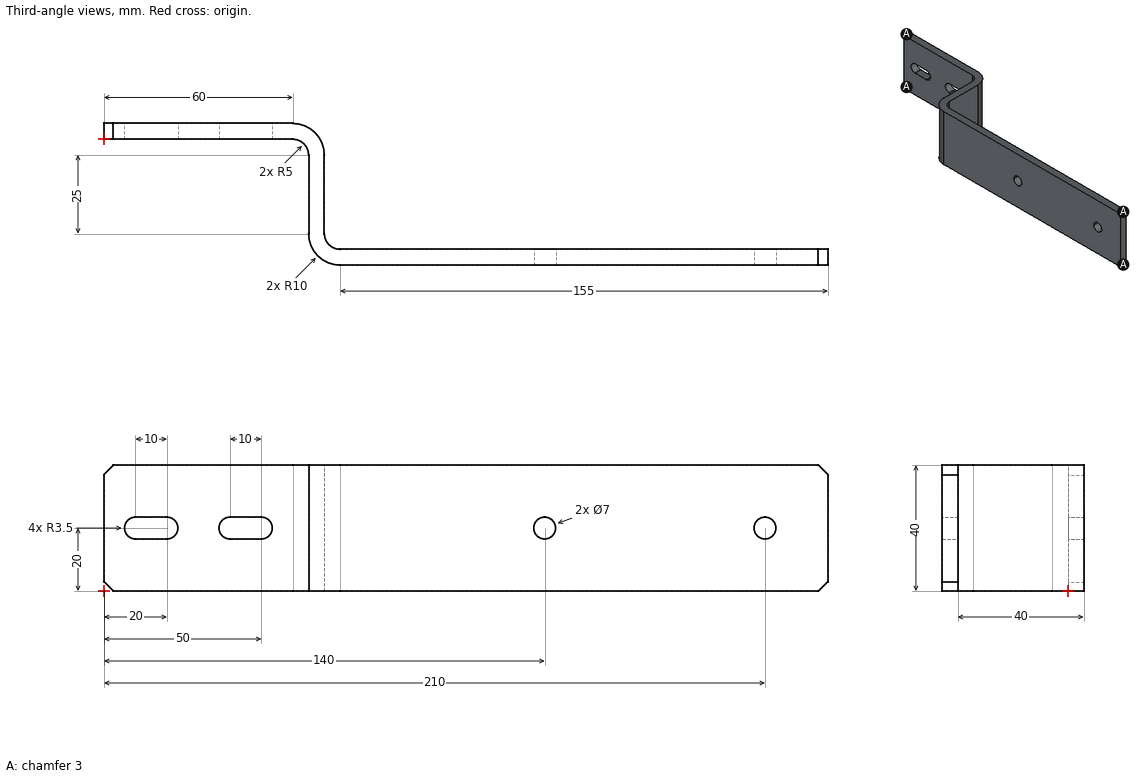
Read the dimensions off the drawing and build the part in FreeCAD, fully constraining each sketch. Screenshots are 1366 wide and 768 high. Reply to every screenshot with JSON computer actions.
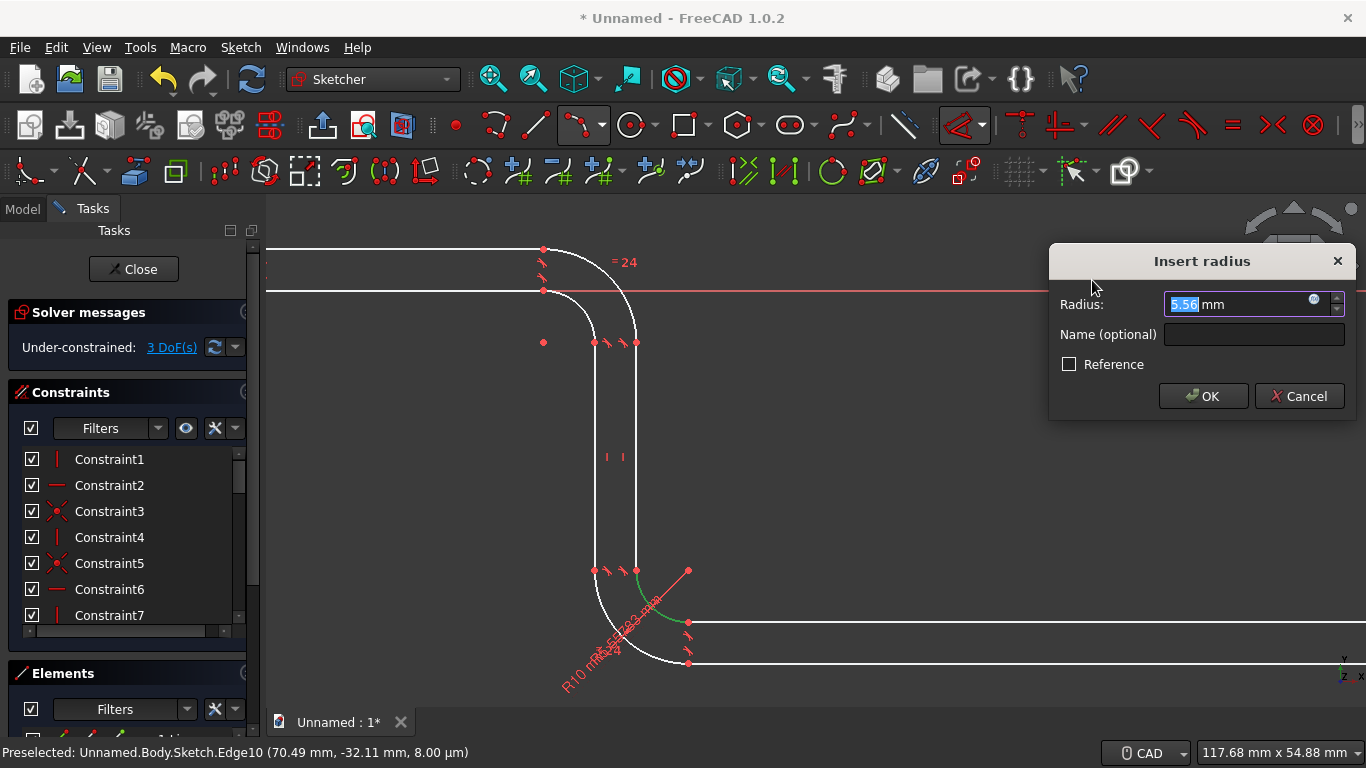
{"action": "type", "text": "5"}
{"action": "key", "text": "Return"}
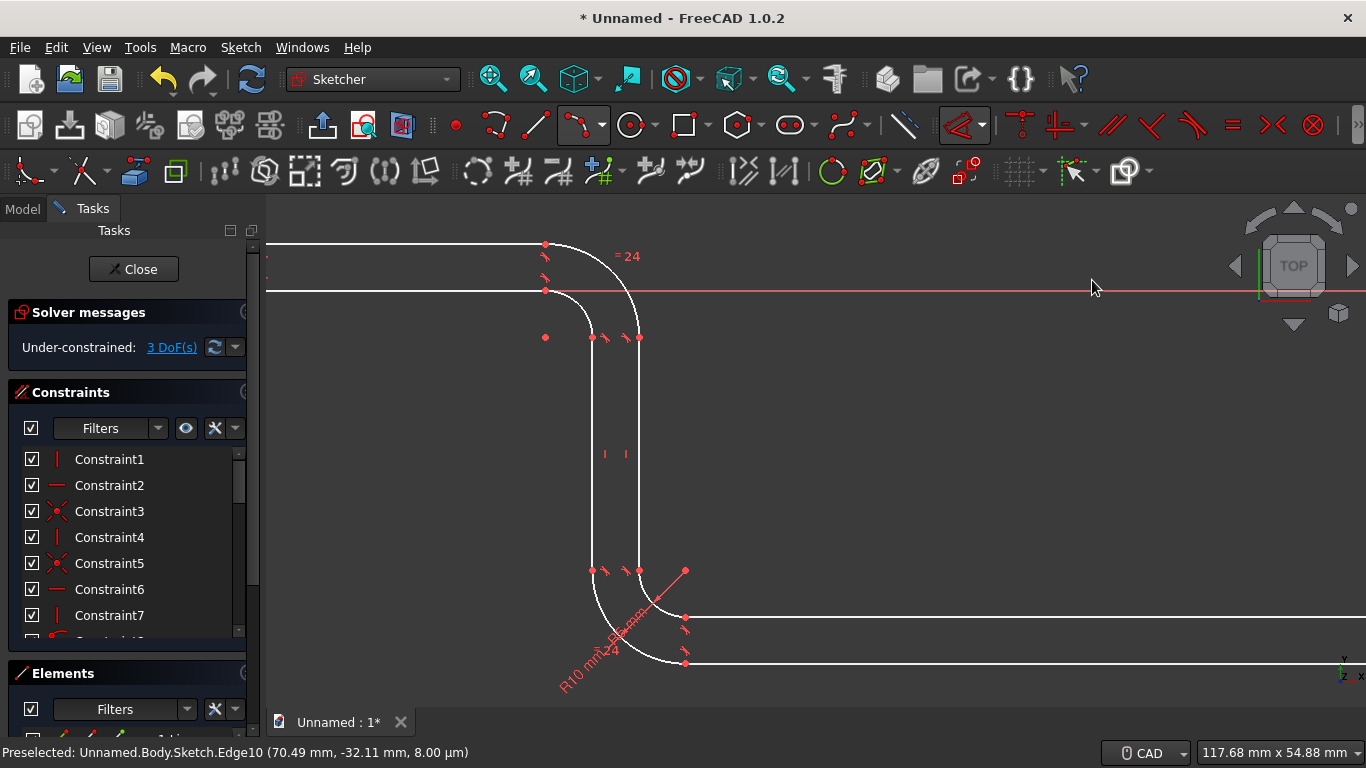
{"action": "scroll", "coordinate": [614, 449], "scroll_direction": "down", "scroll_amount": 6}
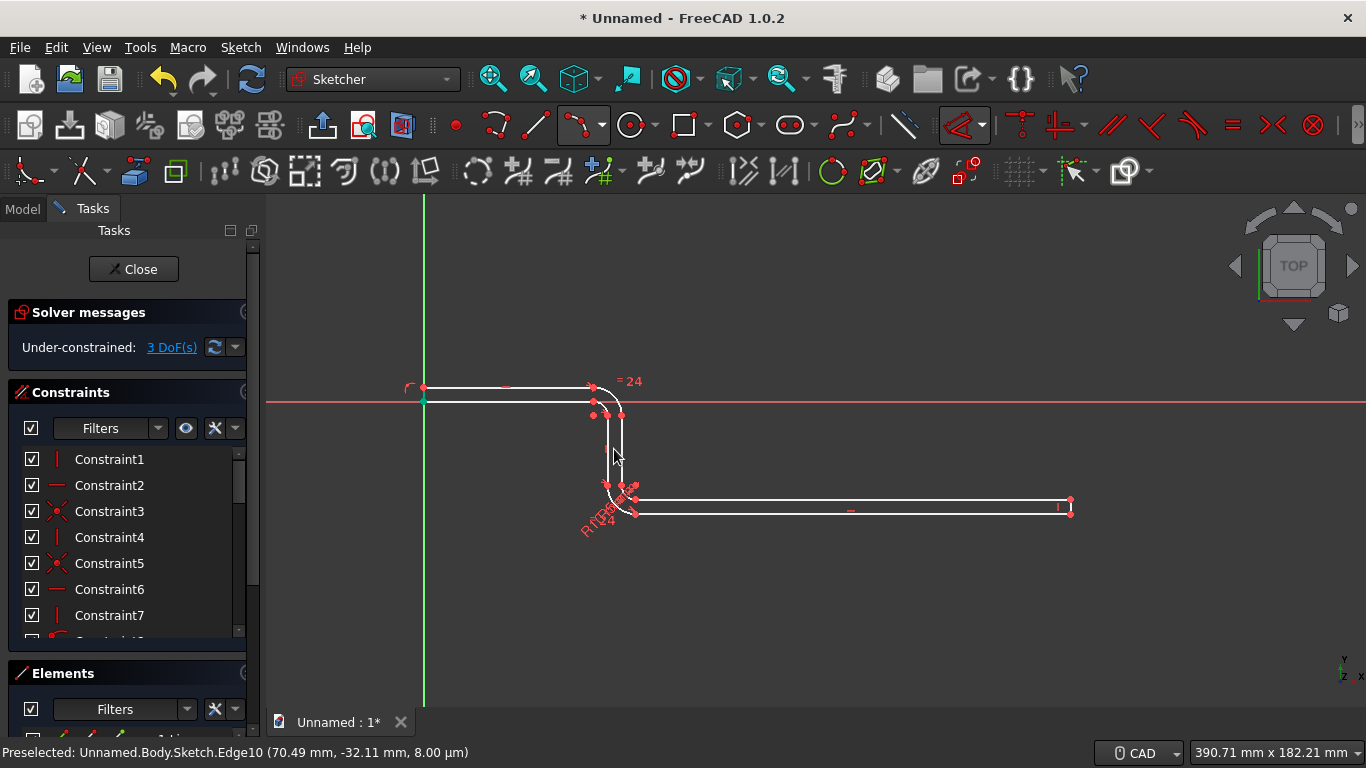
{"action": "left_click", "coordinate": [608, 437]}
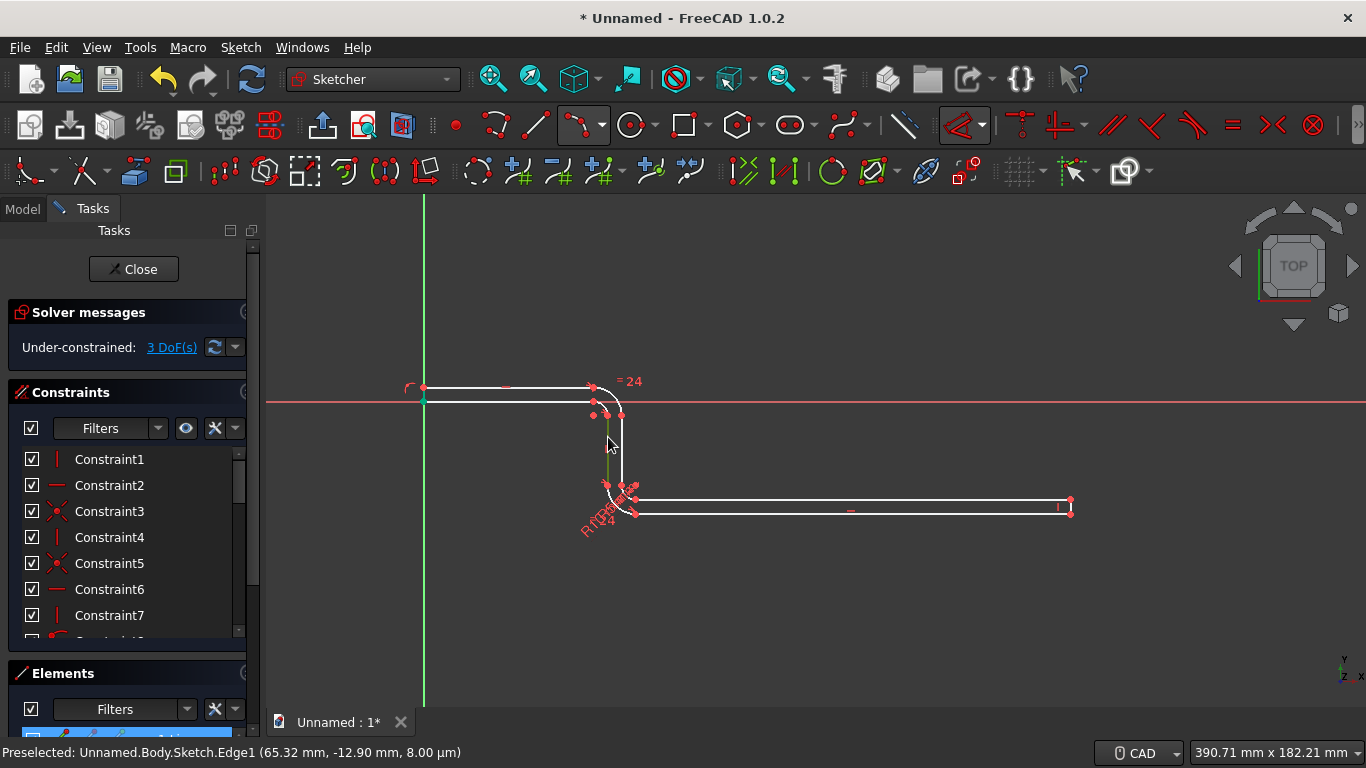
{"action": "key", "text": "i"}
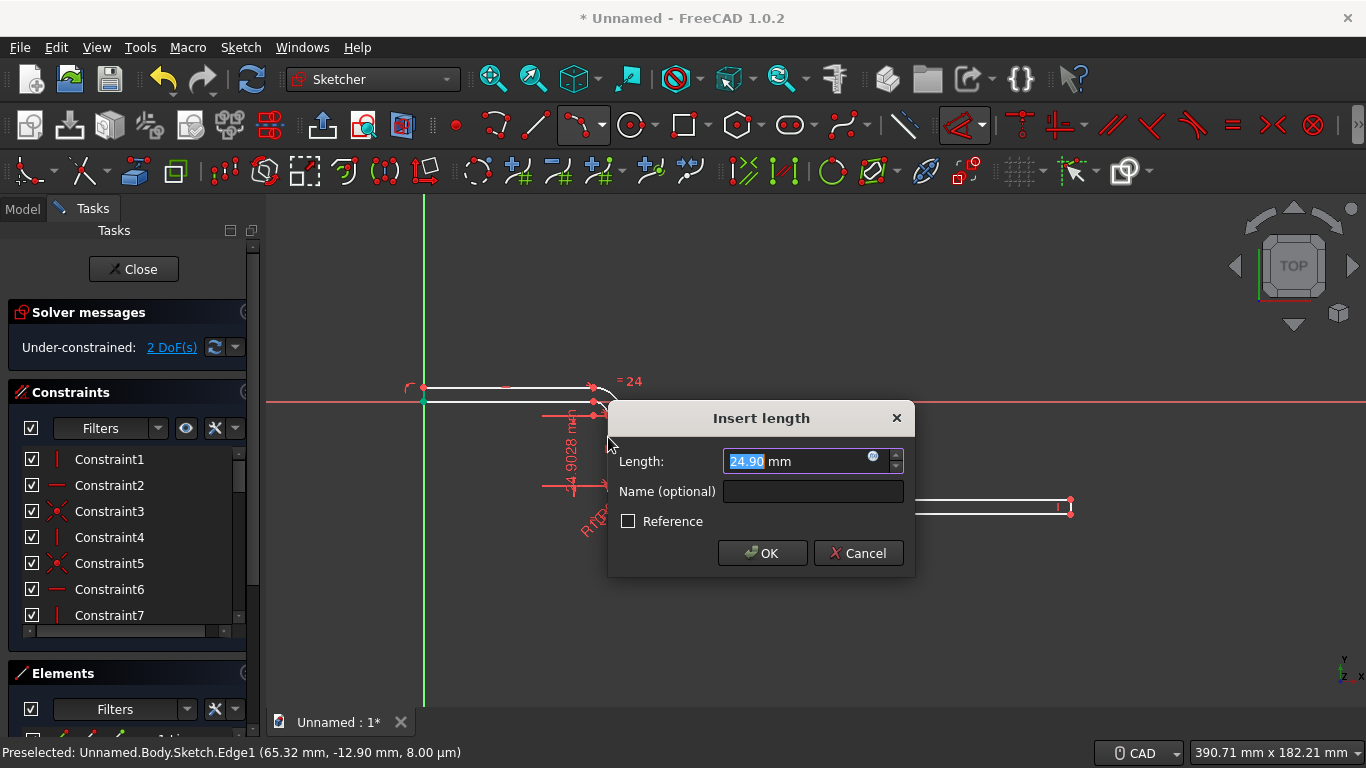
{"action": "type", "text": "25"}
{"action": "key", "text": "Return"}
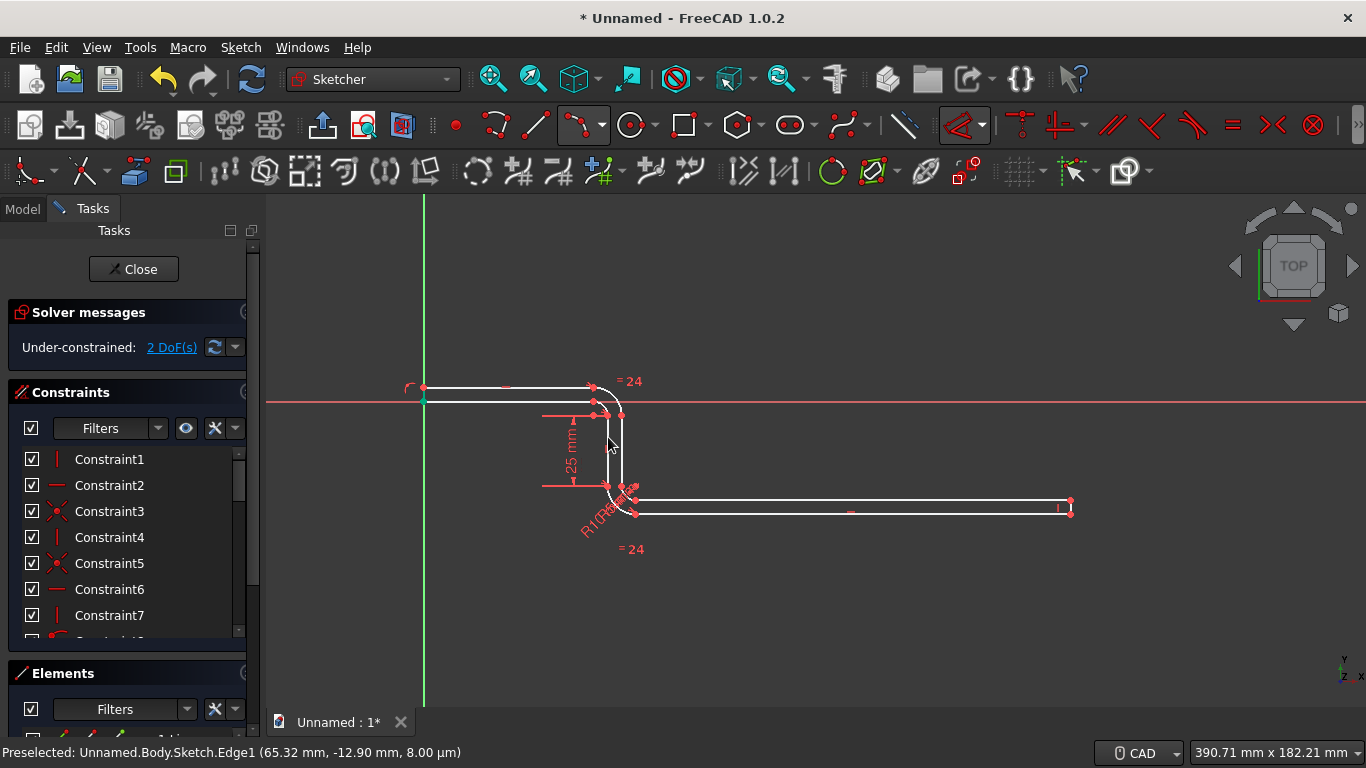
{"action": "left_click", "coordinate": [543, 388]}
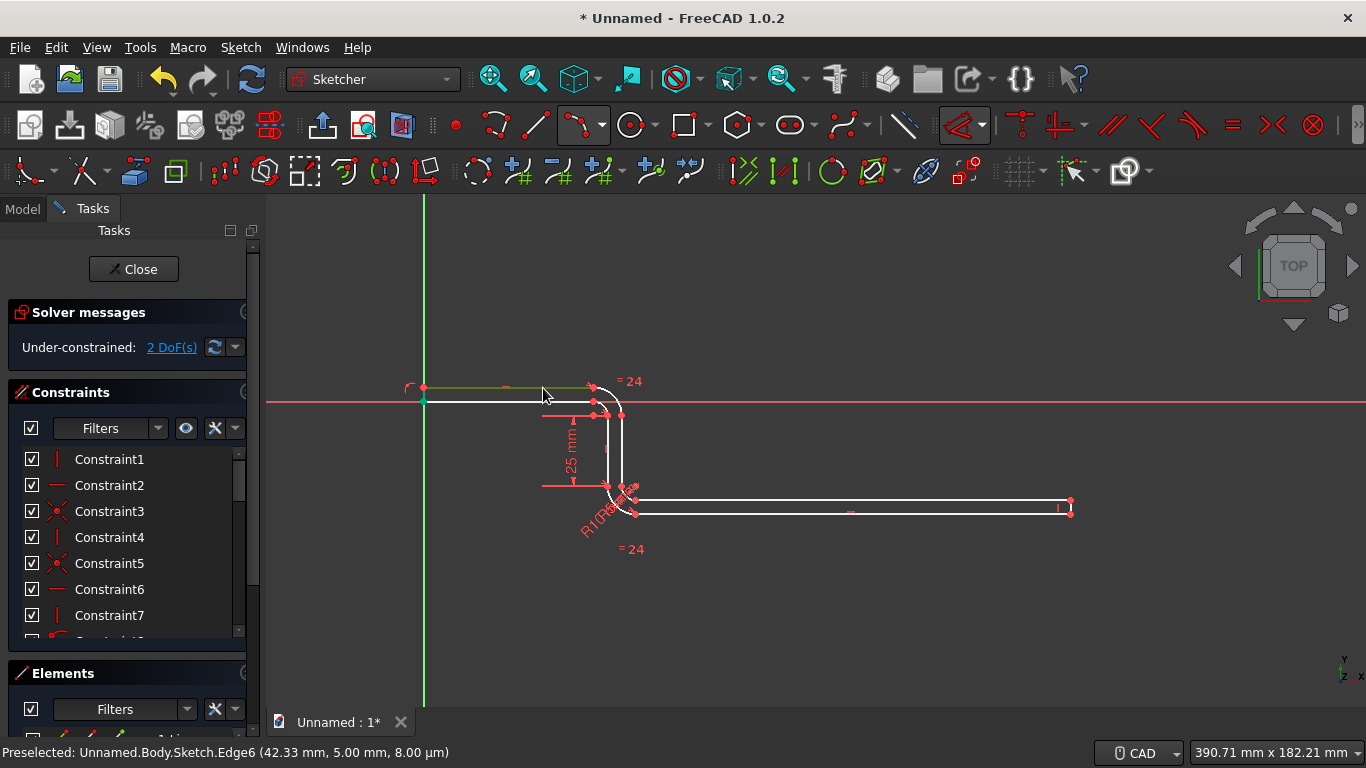
{"action": "key", "text": "l"}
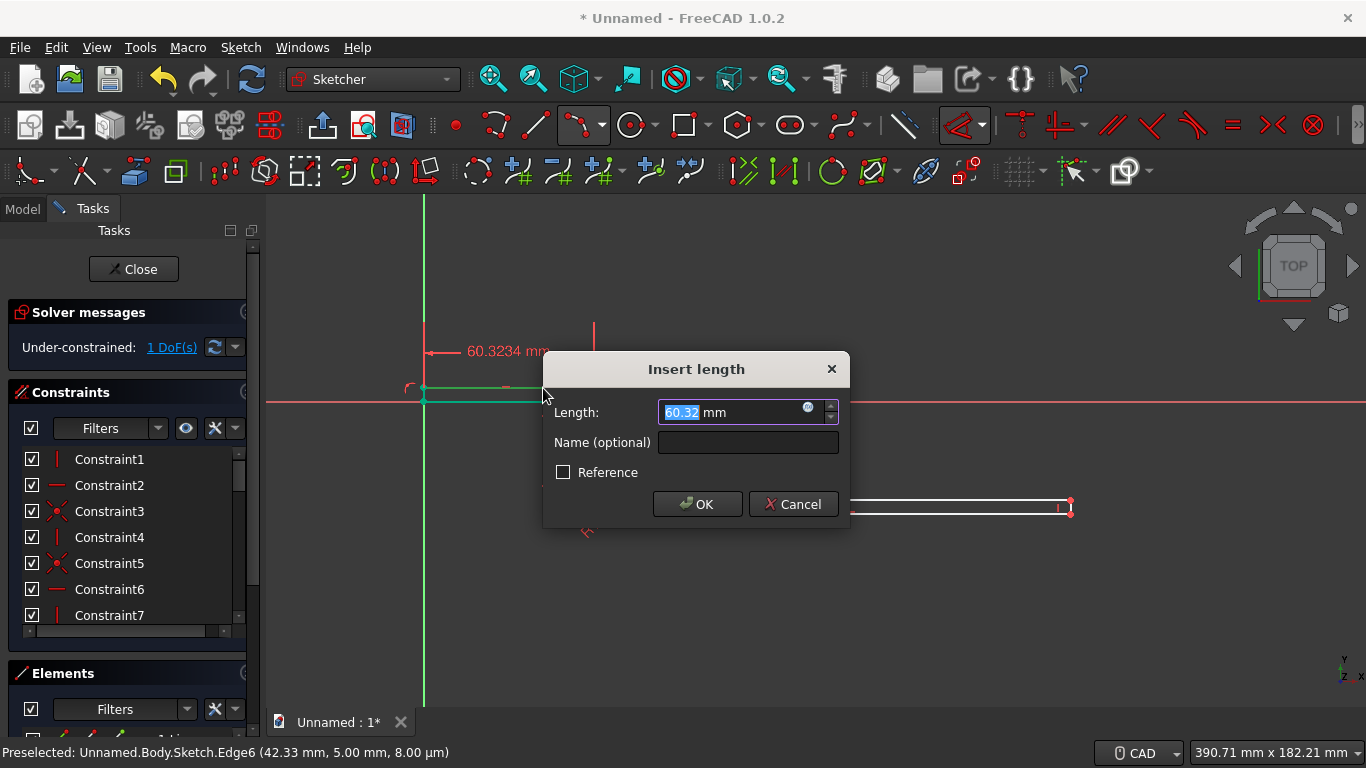
{"action": "type", "text": "60"}
{"action": "key", "text": "Return"}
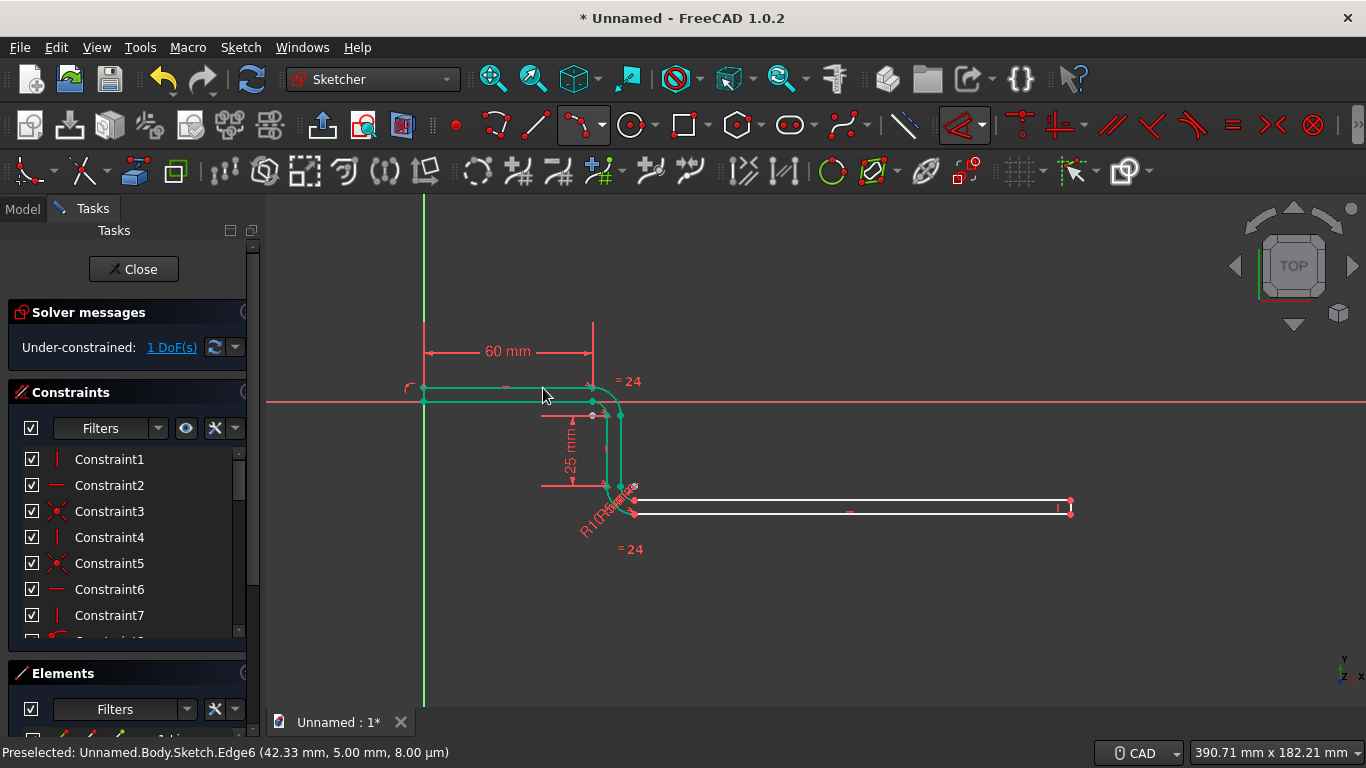
{"action": "left_click", "coordinate": [766, 514]}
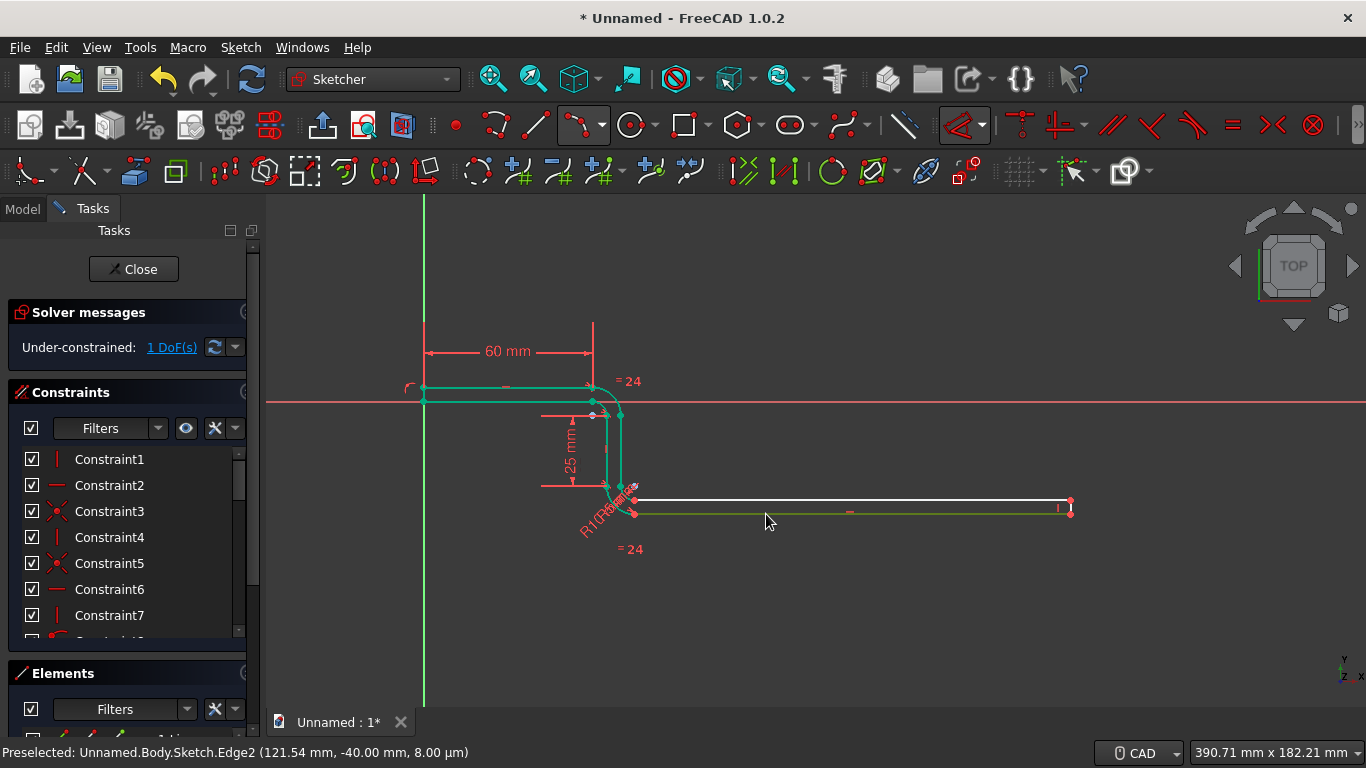
{"action": "key", "text": "l"}